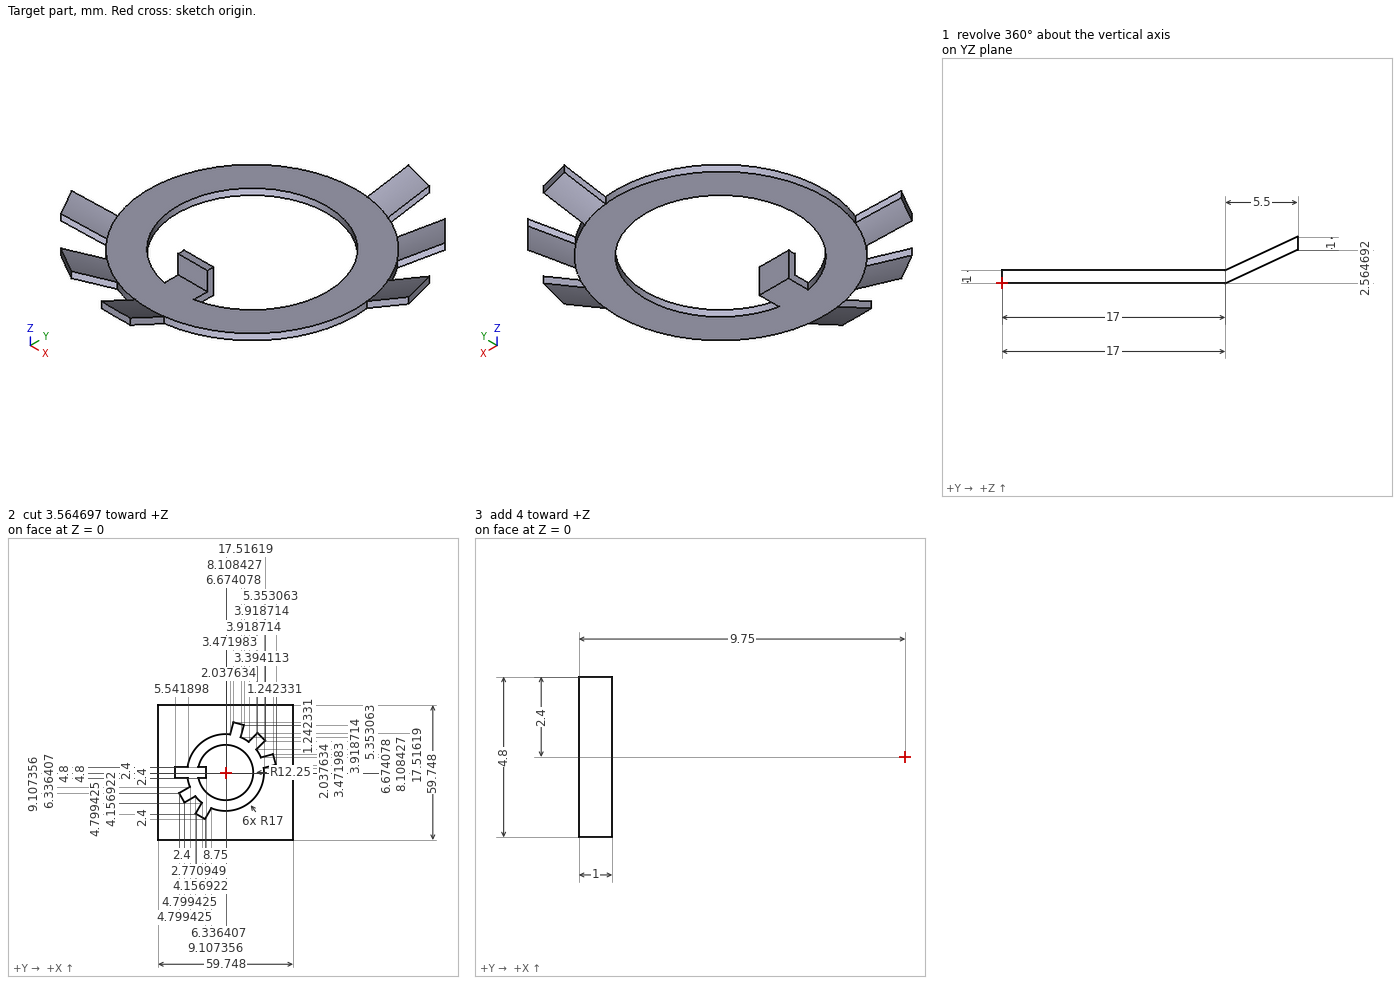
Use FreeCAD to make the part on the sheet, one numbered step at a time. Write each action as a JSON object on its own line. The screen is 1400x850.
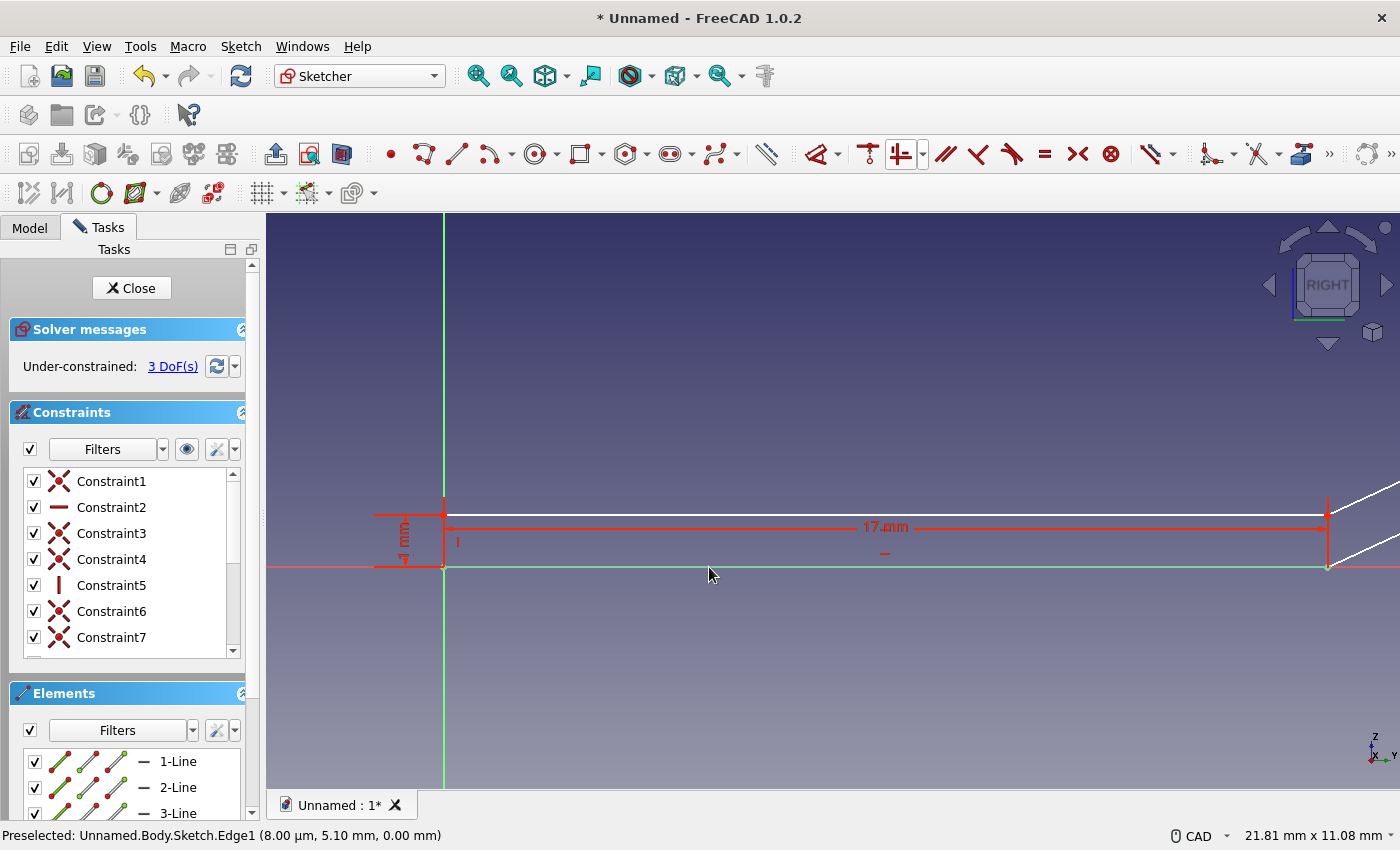
{"action": "left_click", "coordinate": [1062, 515]}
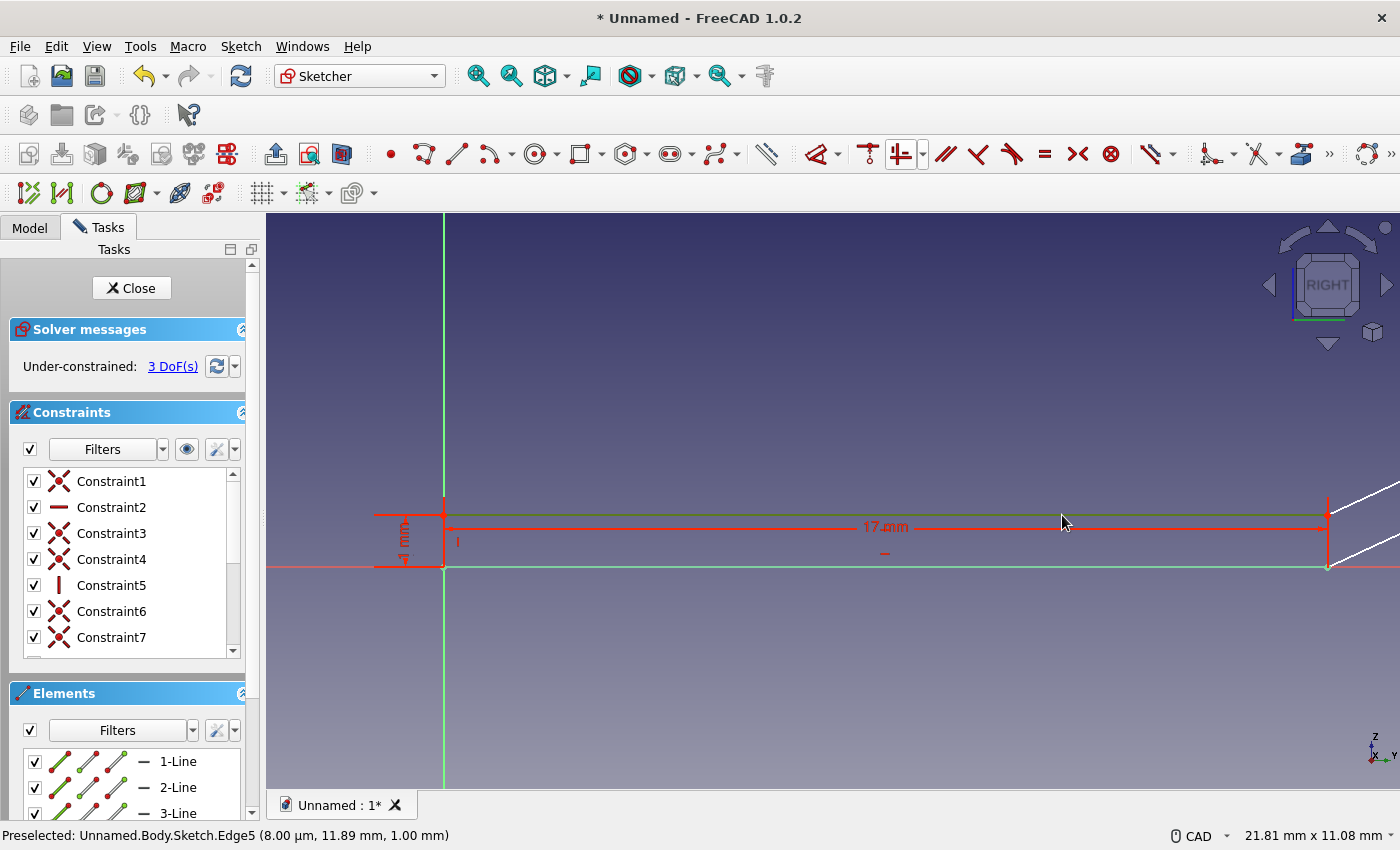
{"action": "left_click", "coordinate": [838, 154]}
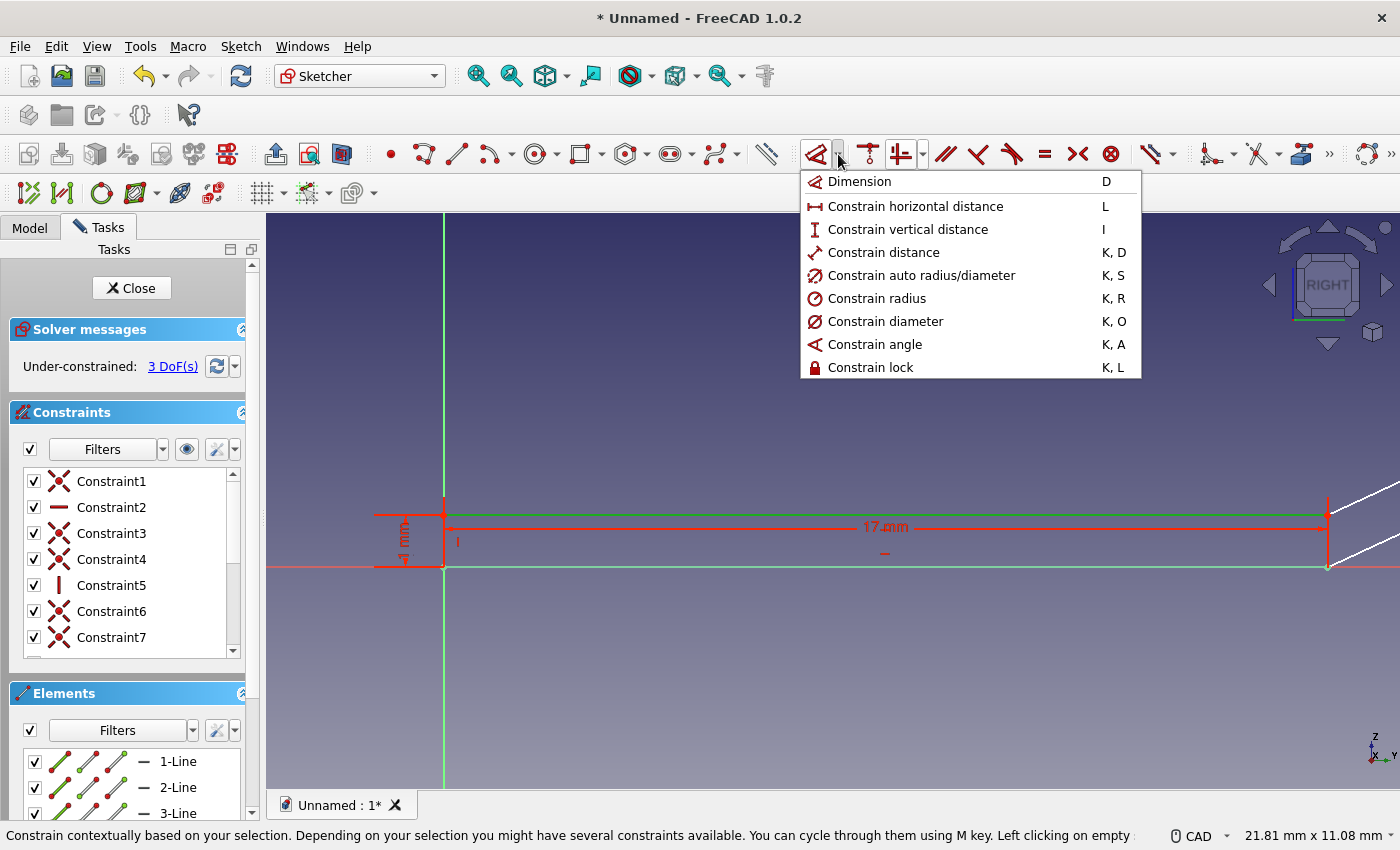
{"action": "left_click", "coordinate": [971, 206]}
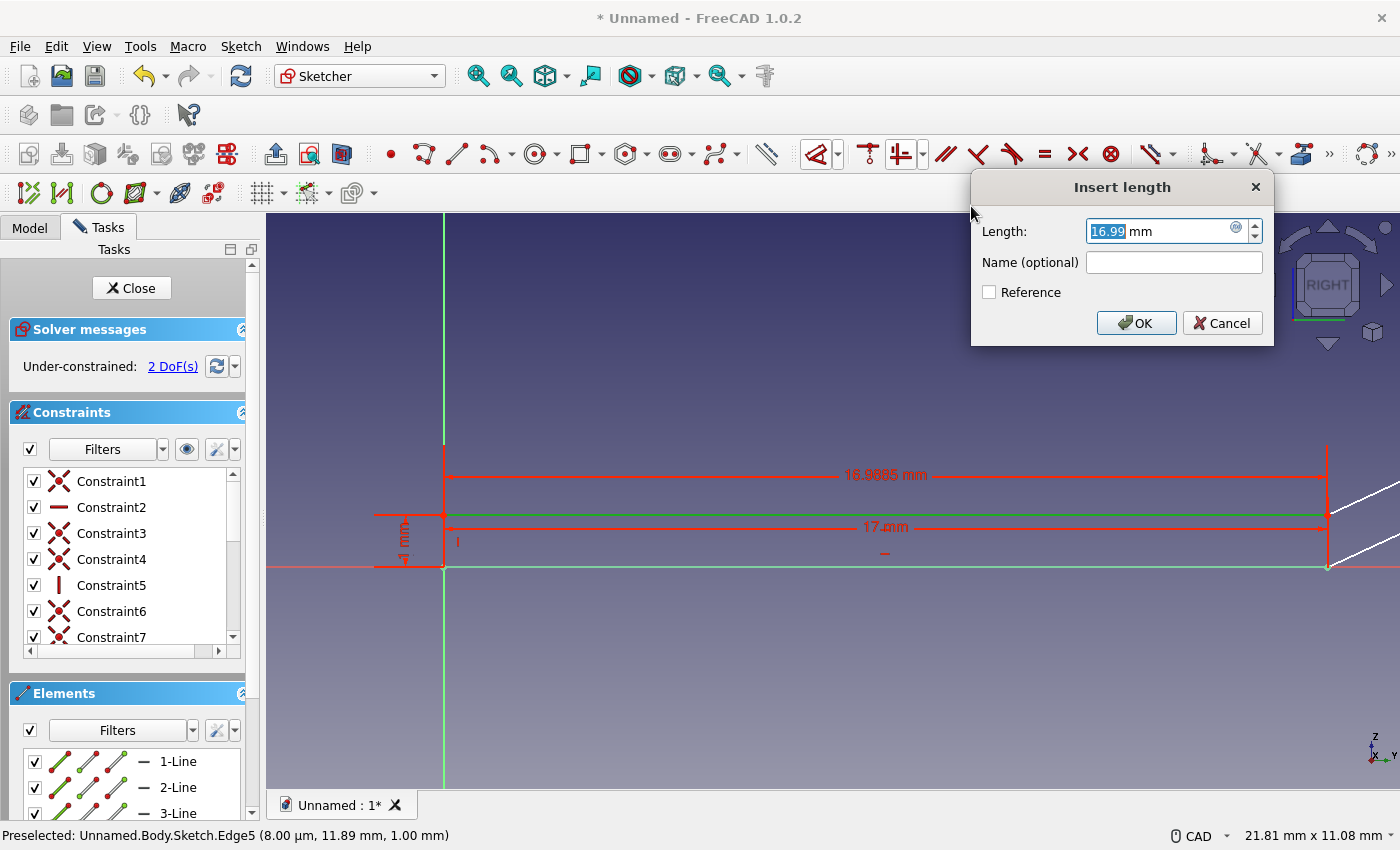
{"action": "type", "text": "17"}
{"action": "key", "text": "Return"}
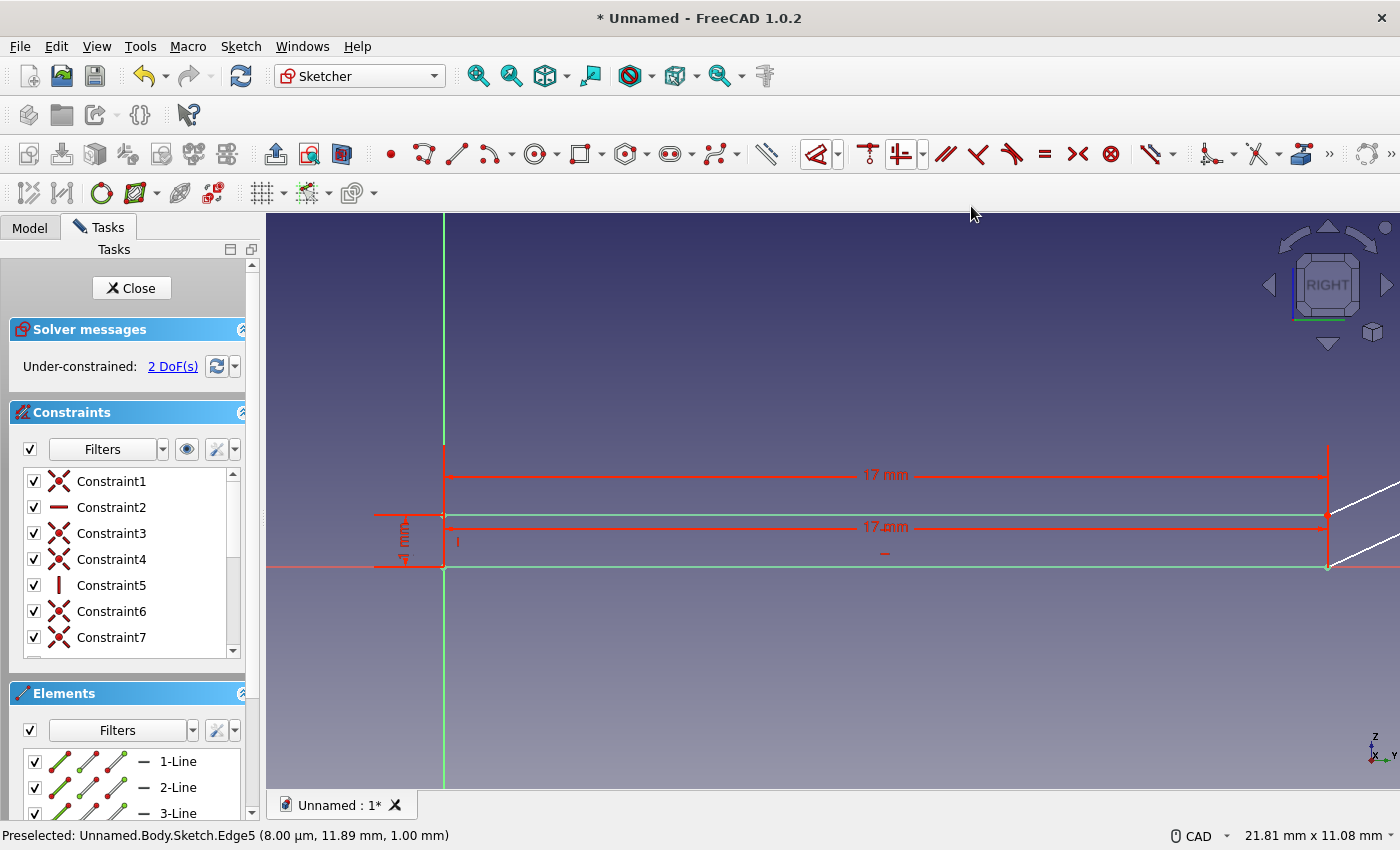
{"action": "scroll", "coordinate": [443, 533], "scroll_direction": "down", "scroll_amount": 3}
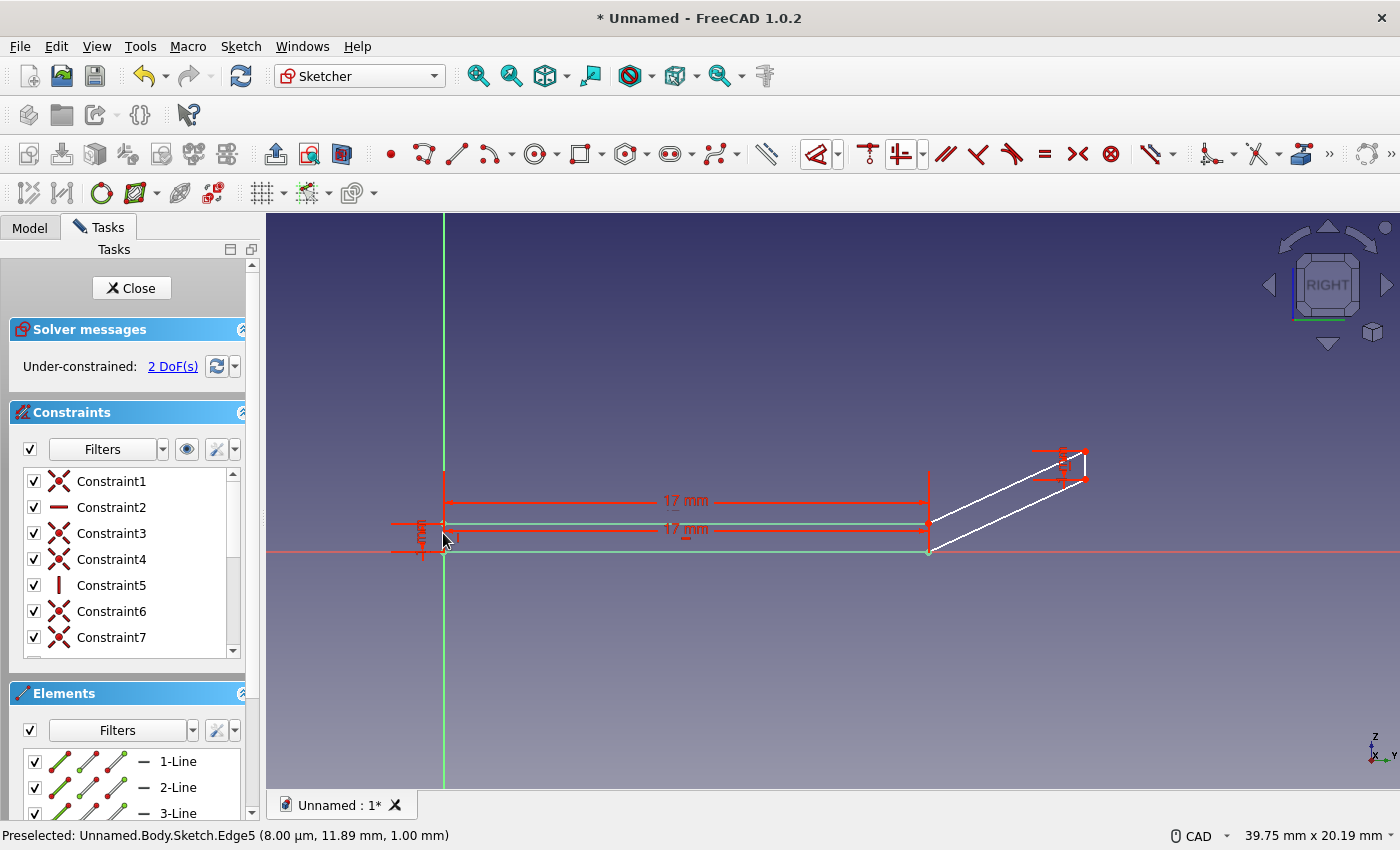
{"action": "left_click", "coordinate": [976, 530]}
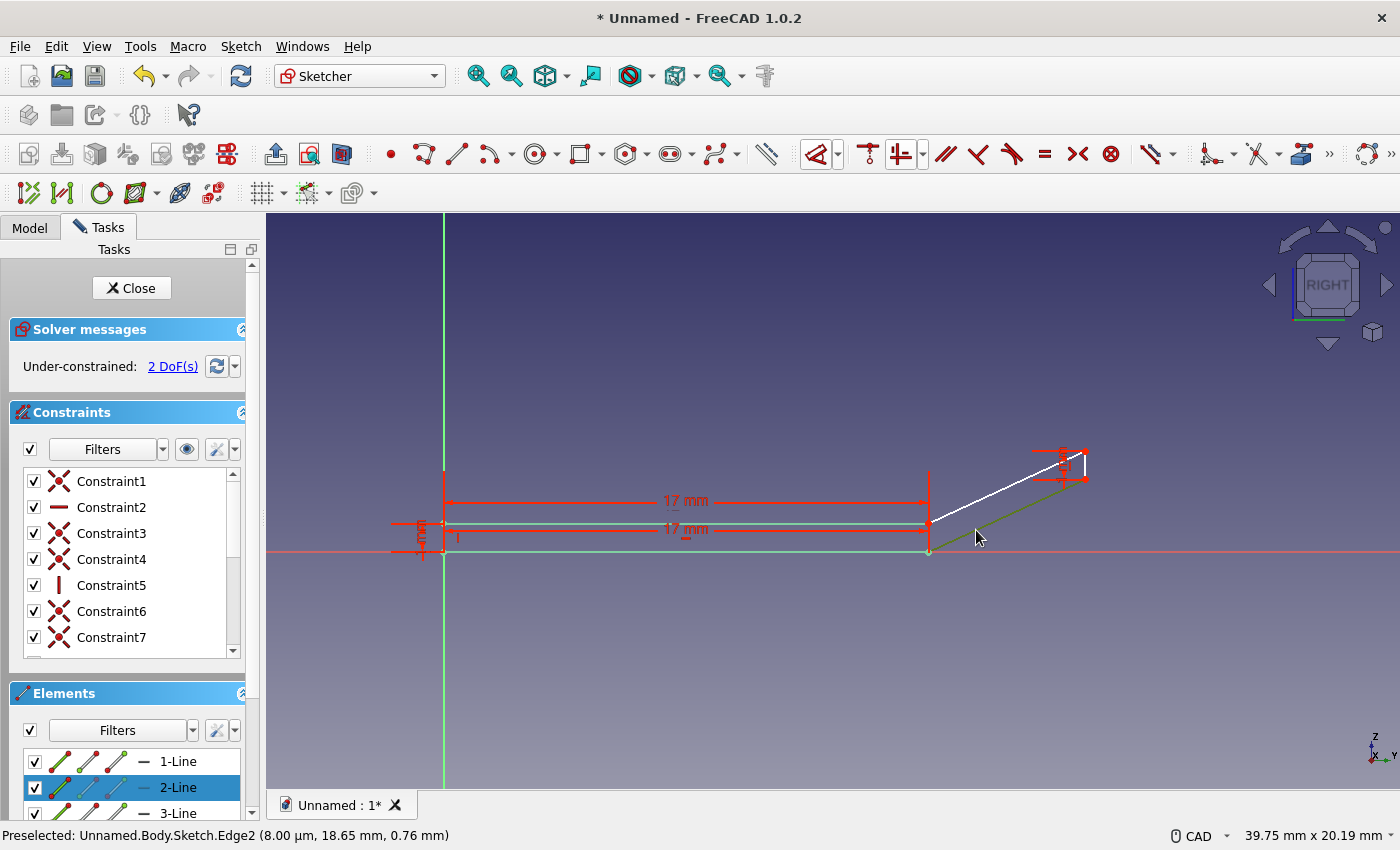
{"action": "left_click", "coordinate": [838, 154]}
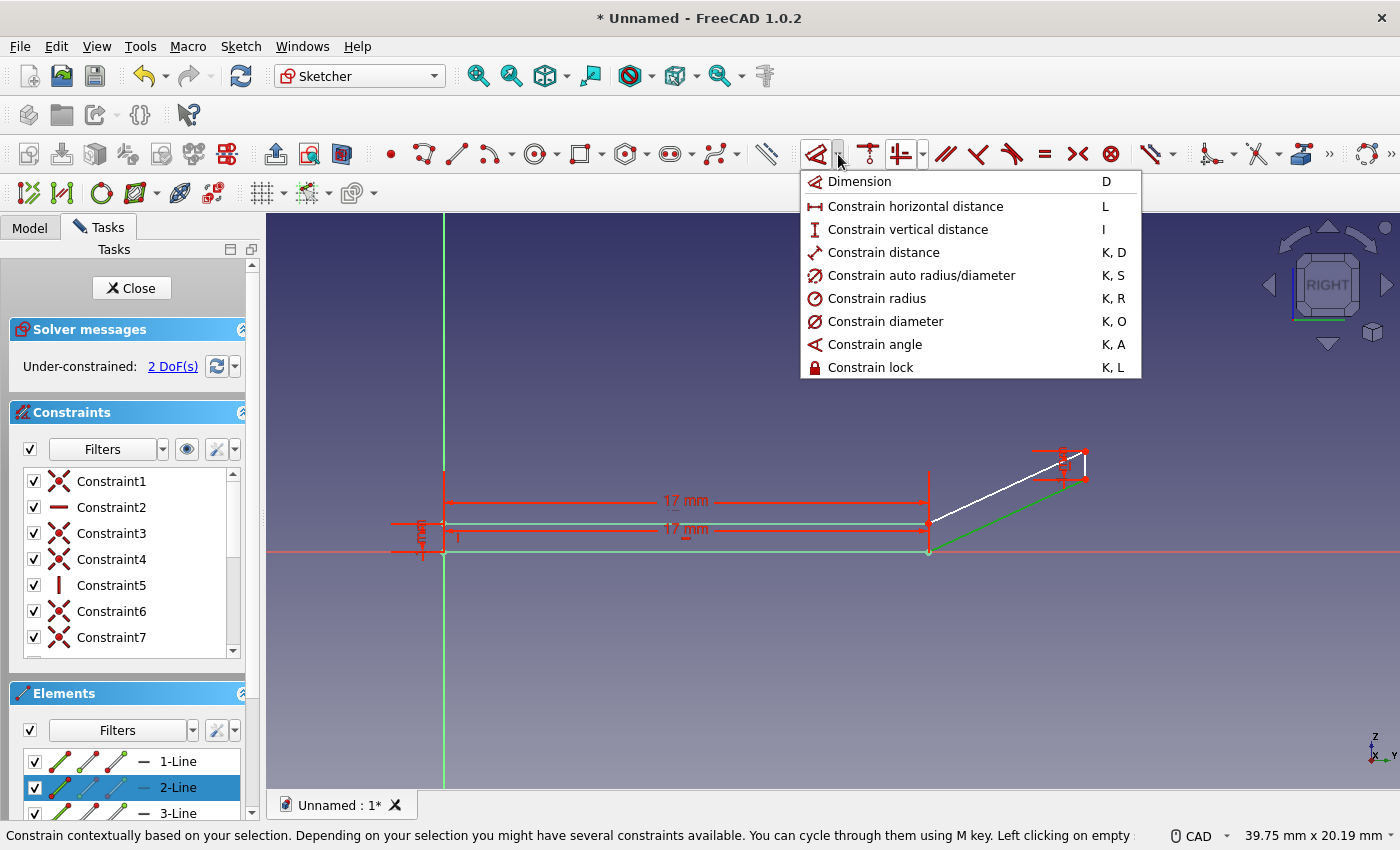
{"action": "left_click", "coordinate": [971, 206]}